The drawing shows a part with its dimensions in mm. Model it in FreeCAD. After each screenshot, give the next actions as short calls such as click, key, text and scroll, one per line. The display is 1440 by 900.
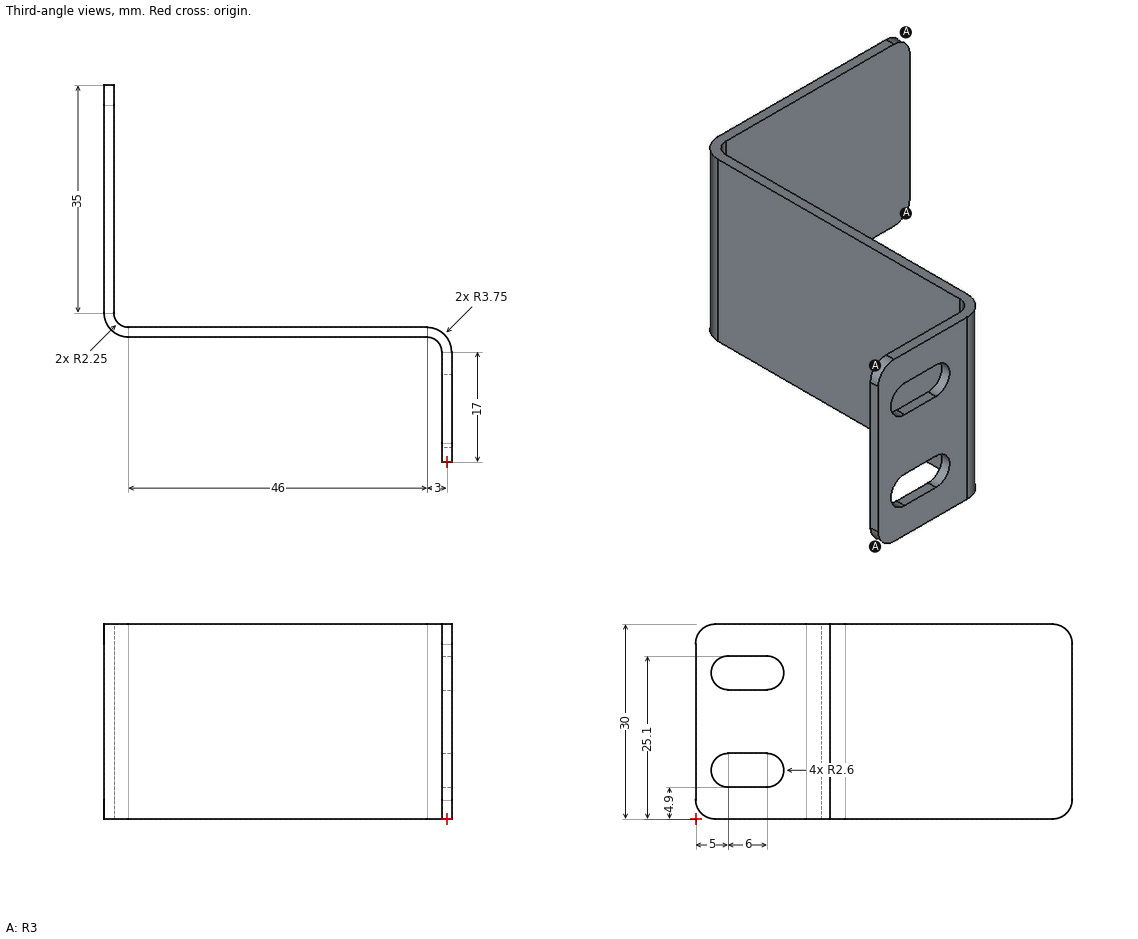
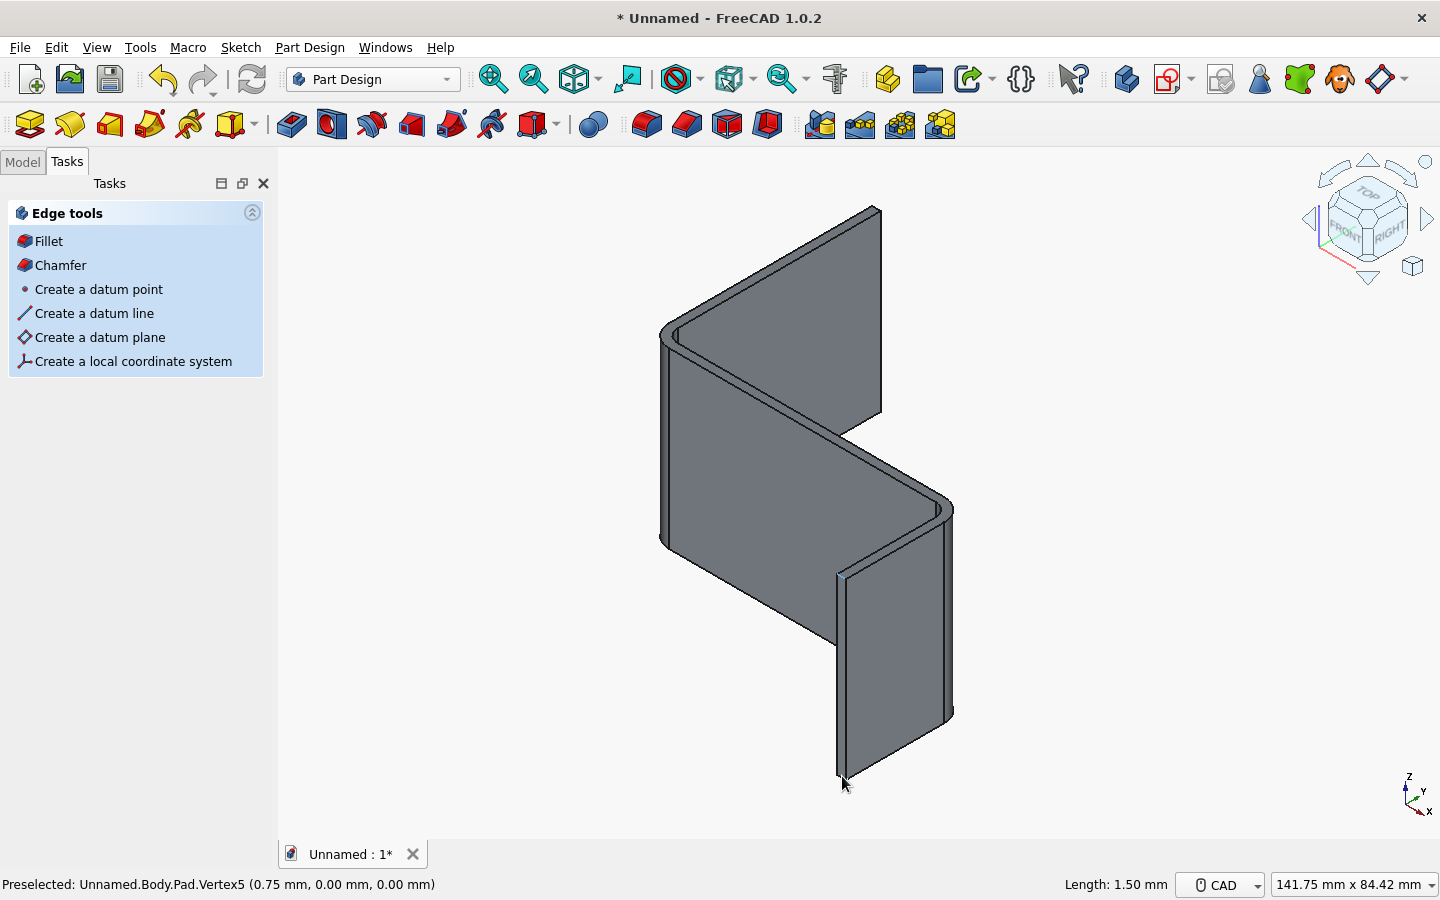
key(2)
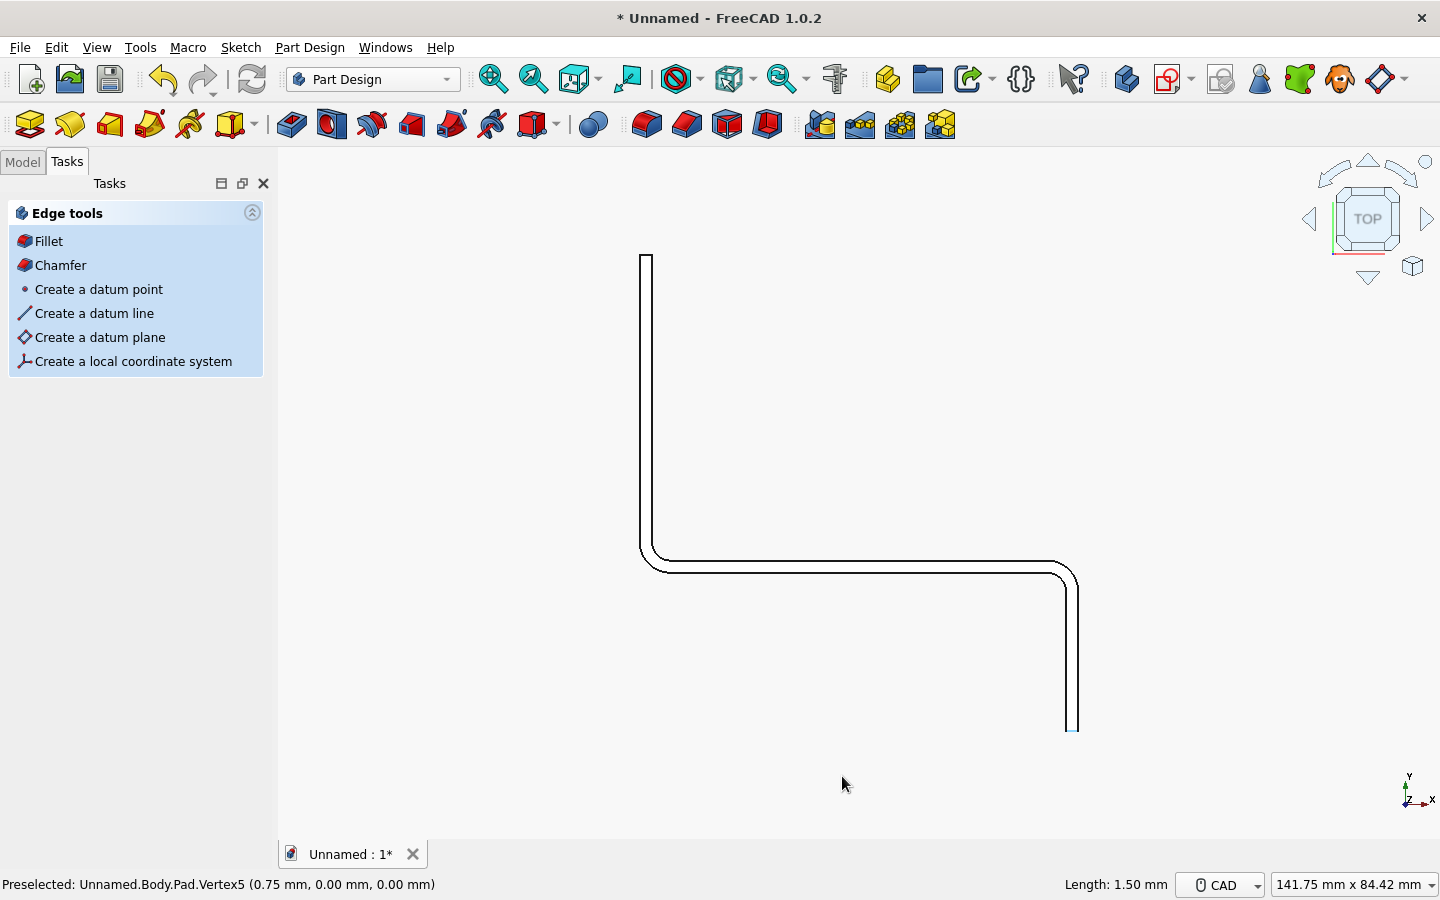
click(646, 254, ctrl)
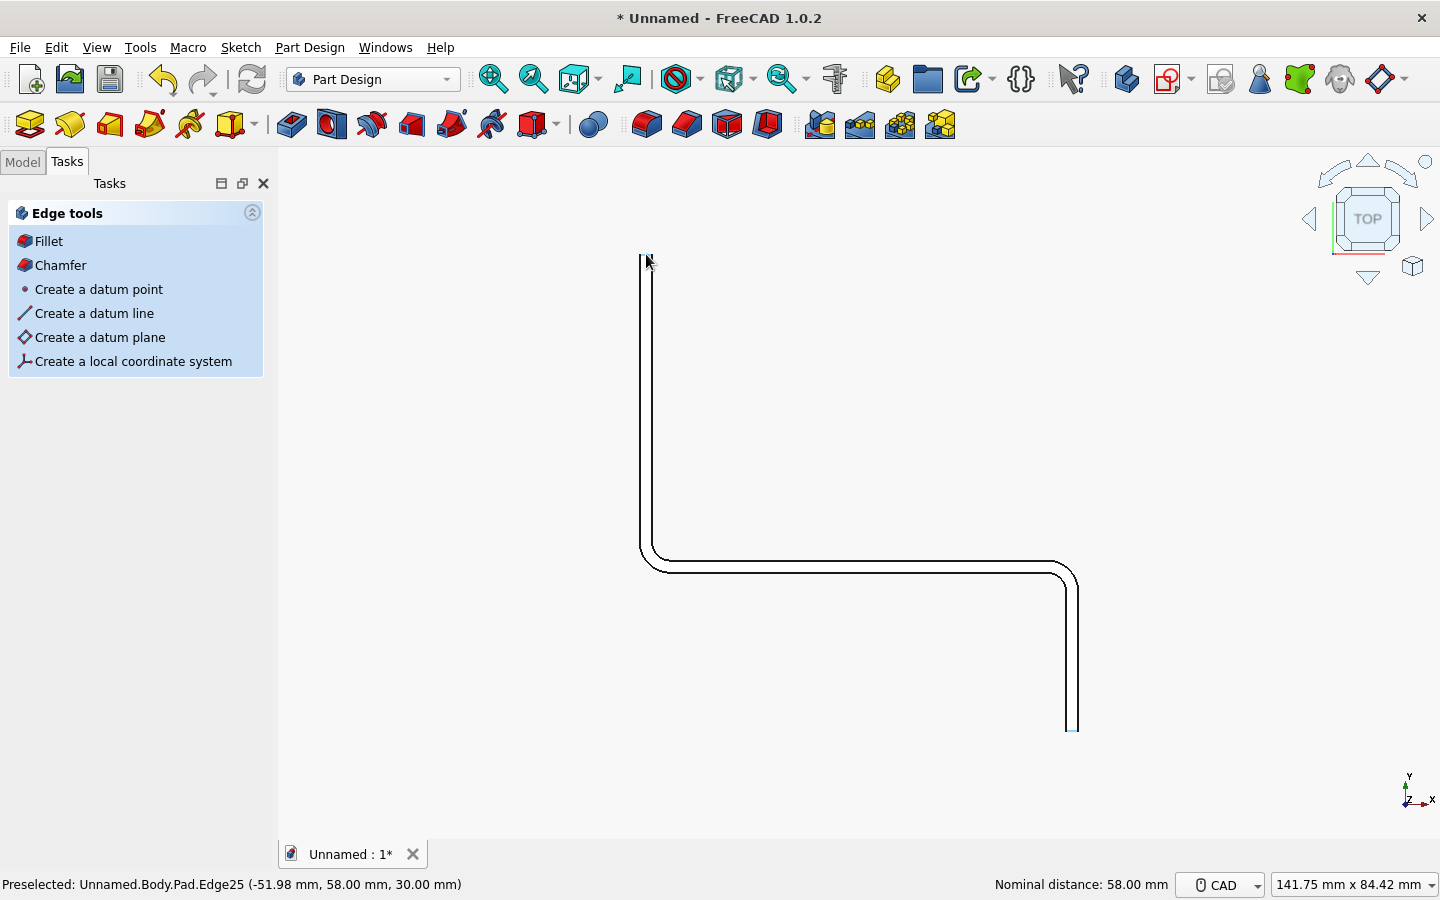
scroll(1072, 730, up, 6)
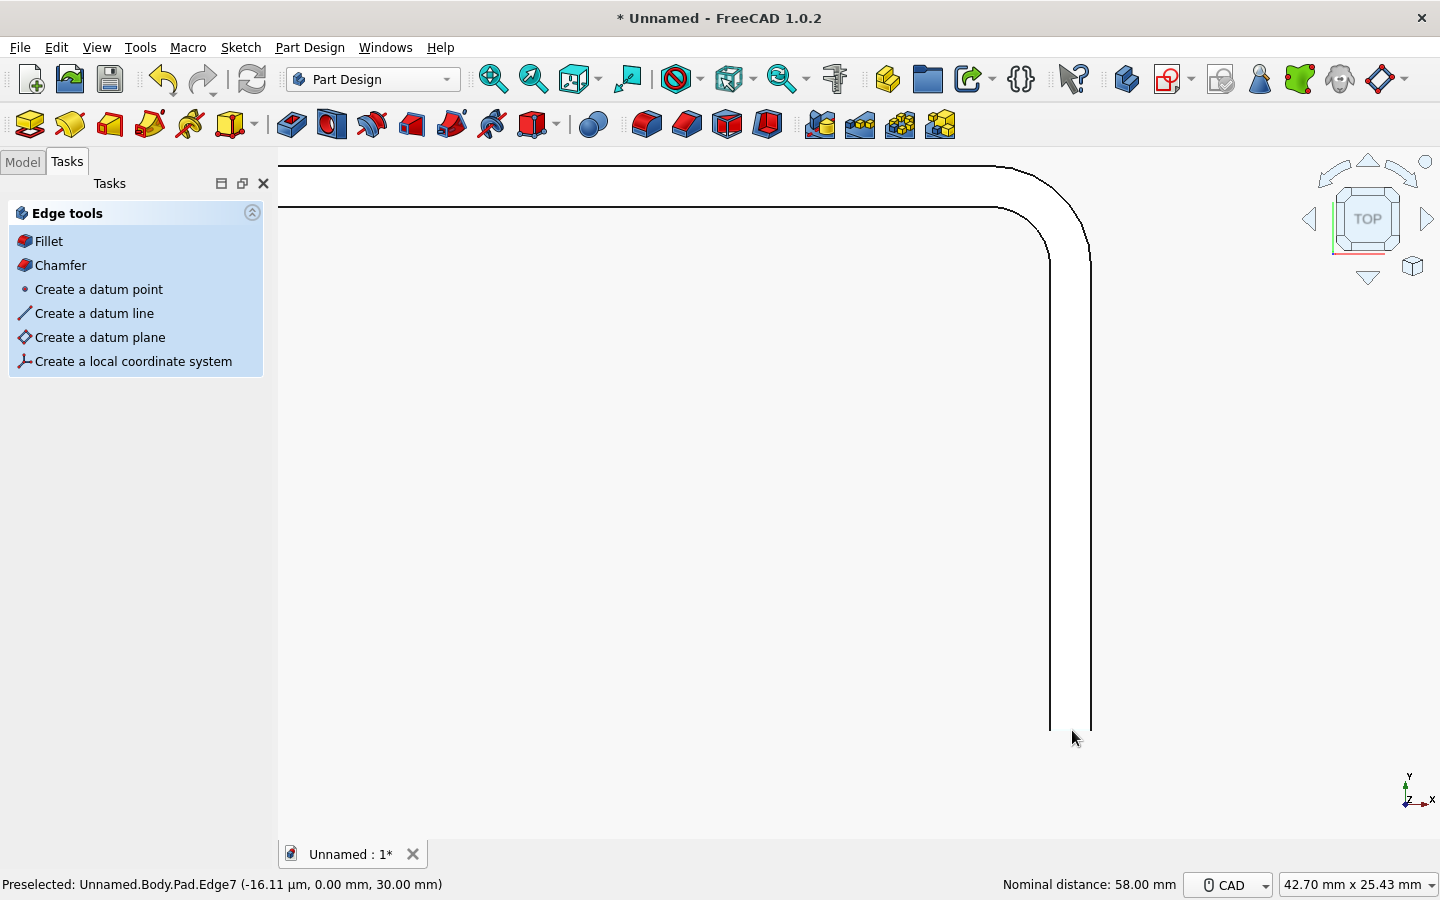
click(494, 80)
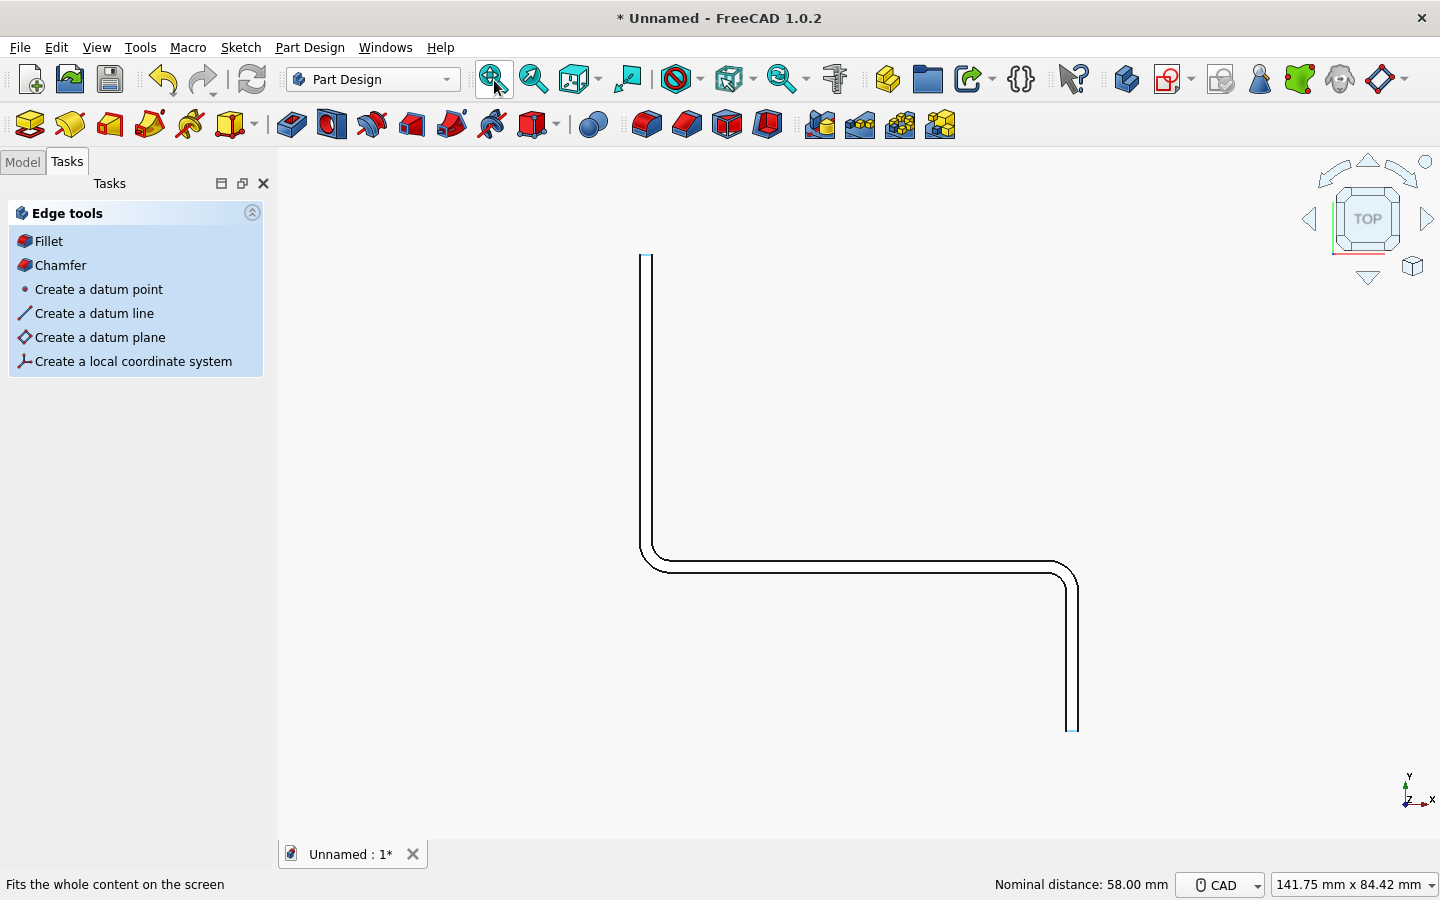
key(1)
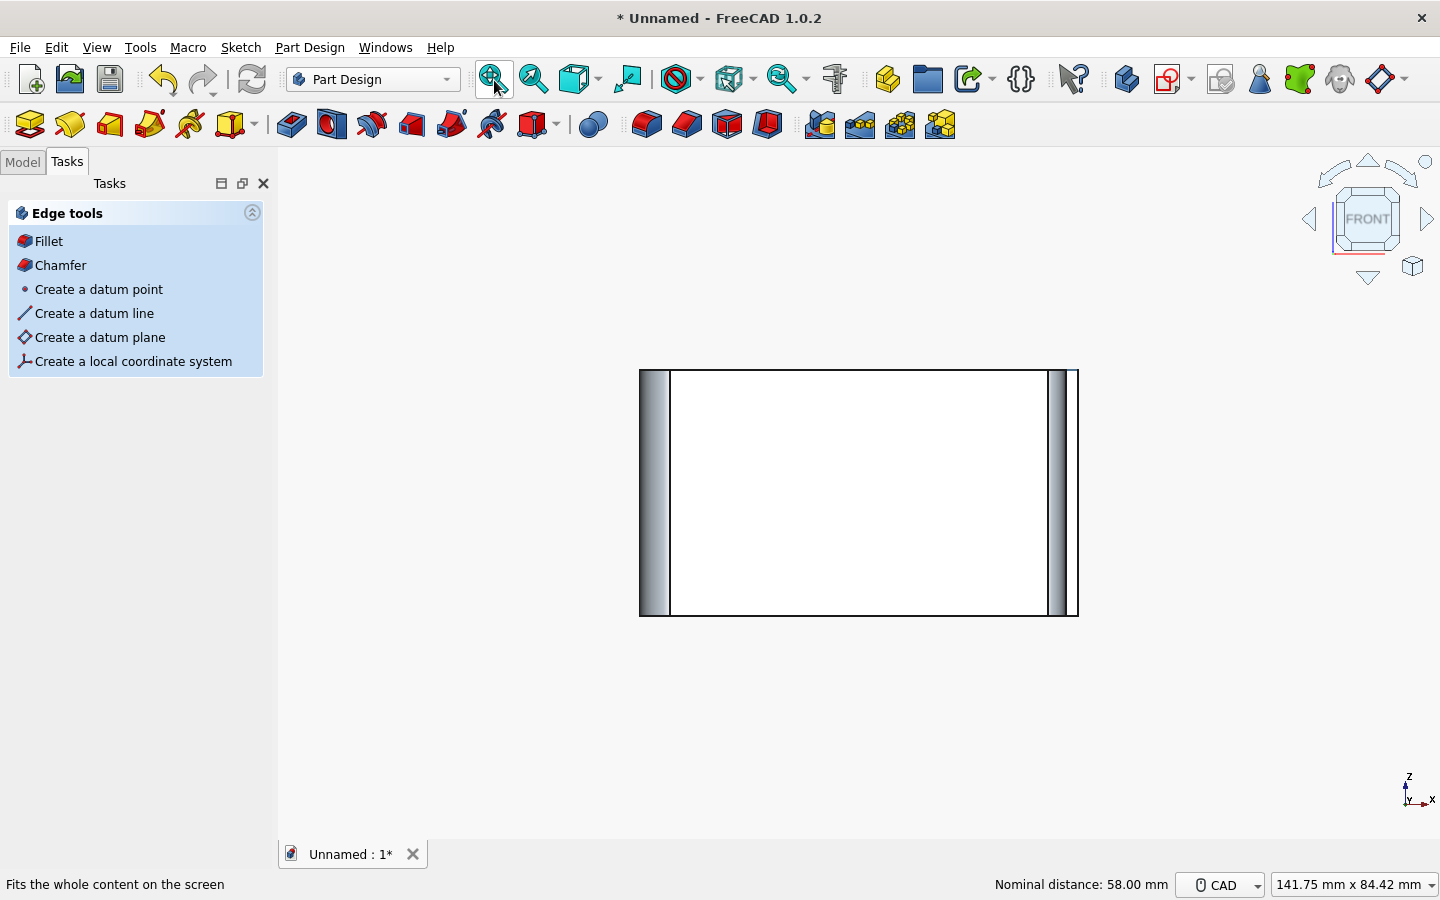
click(494, 80)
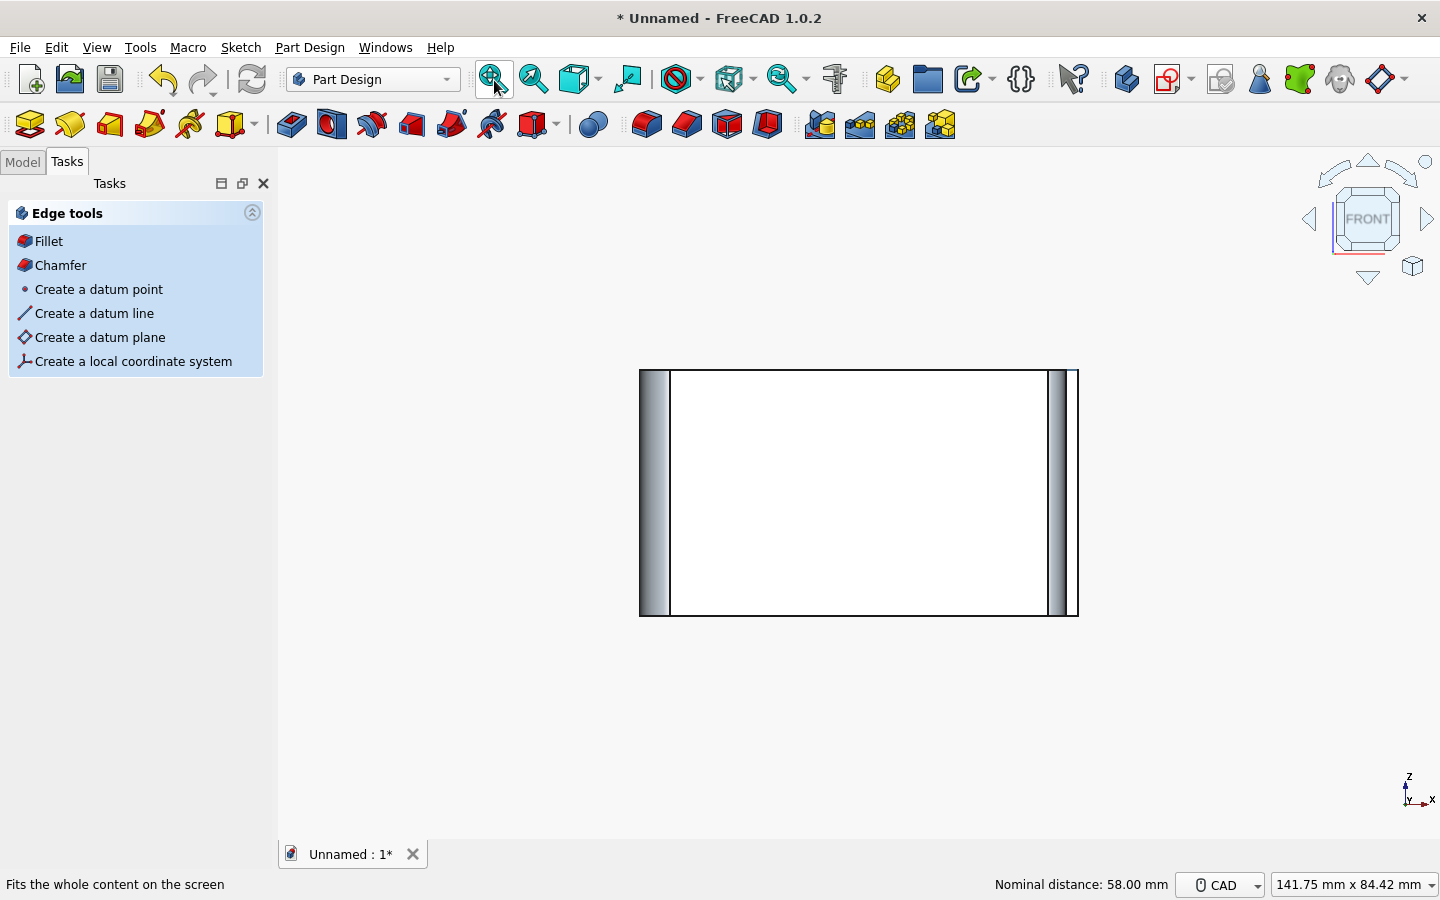
click(1072, 615, ctrl)